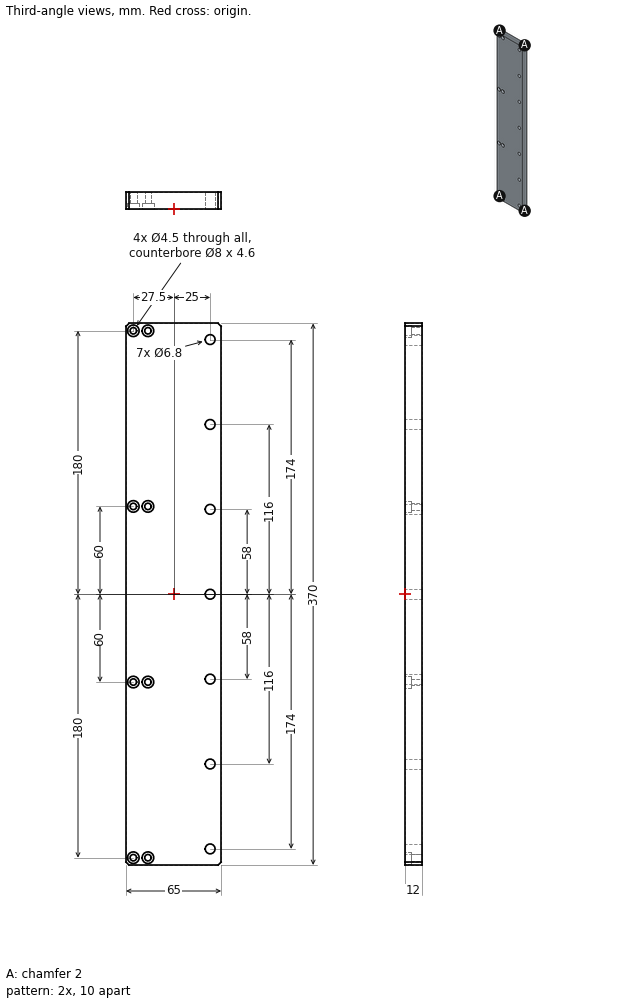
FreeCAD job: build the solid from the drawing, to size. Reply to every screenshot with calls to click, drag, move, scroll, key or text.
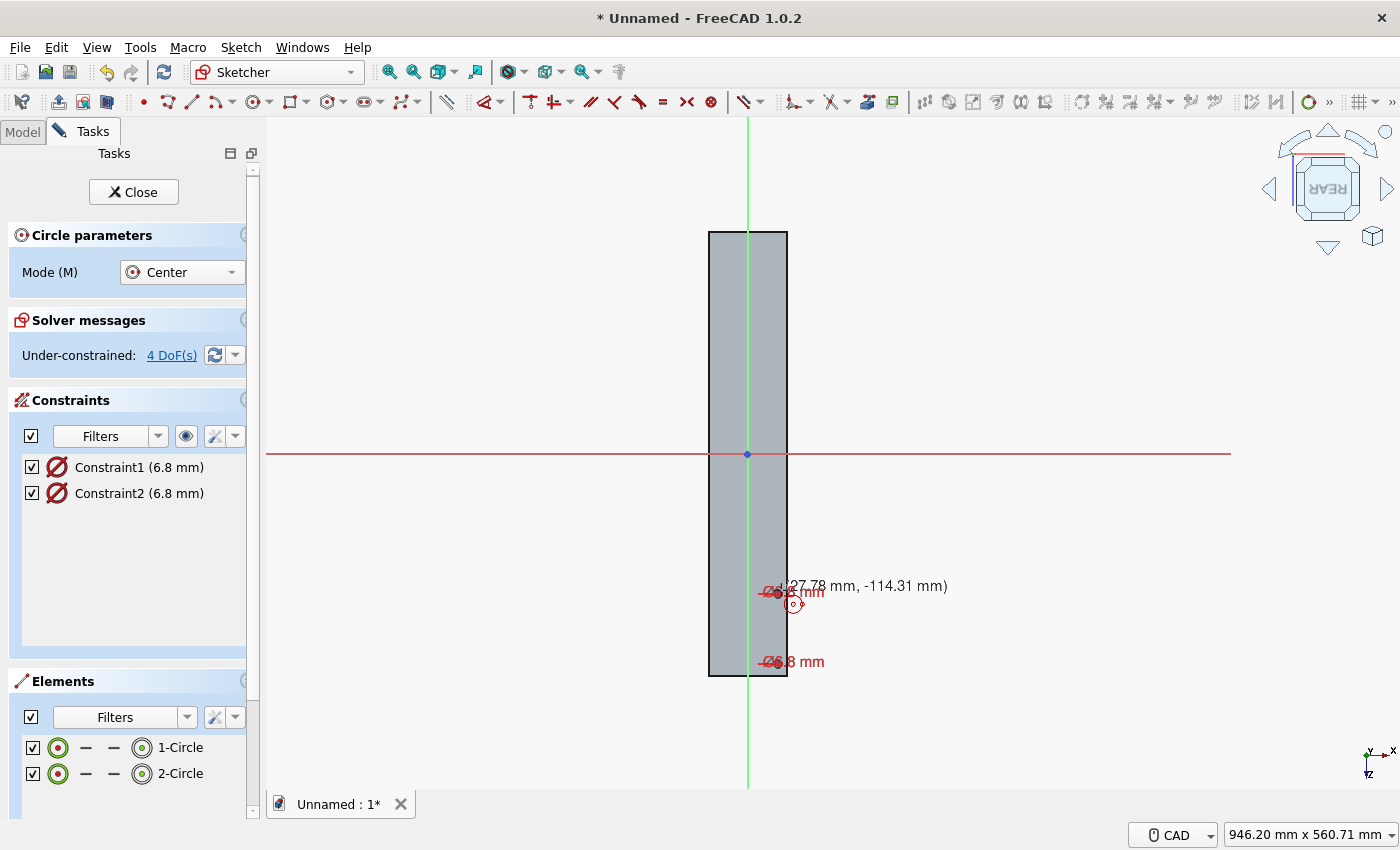
scroll(778, 524, up, 9)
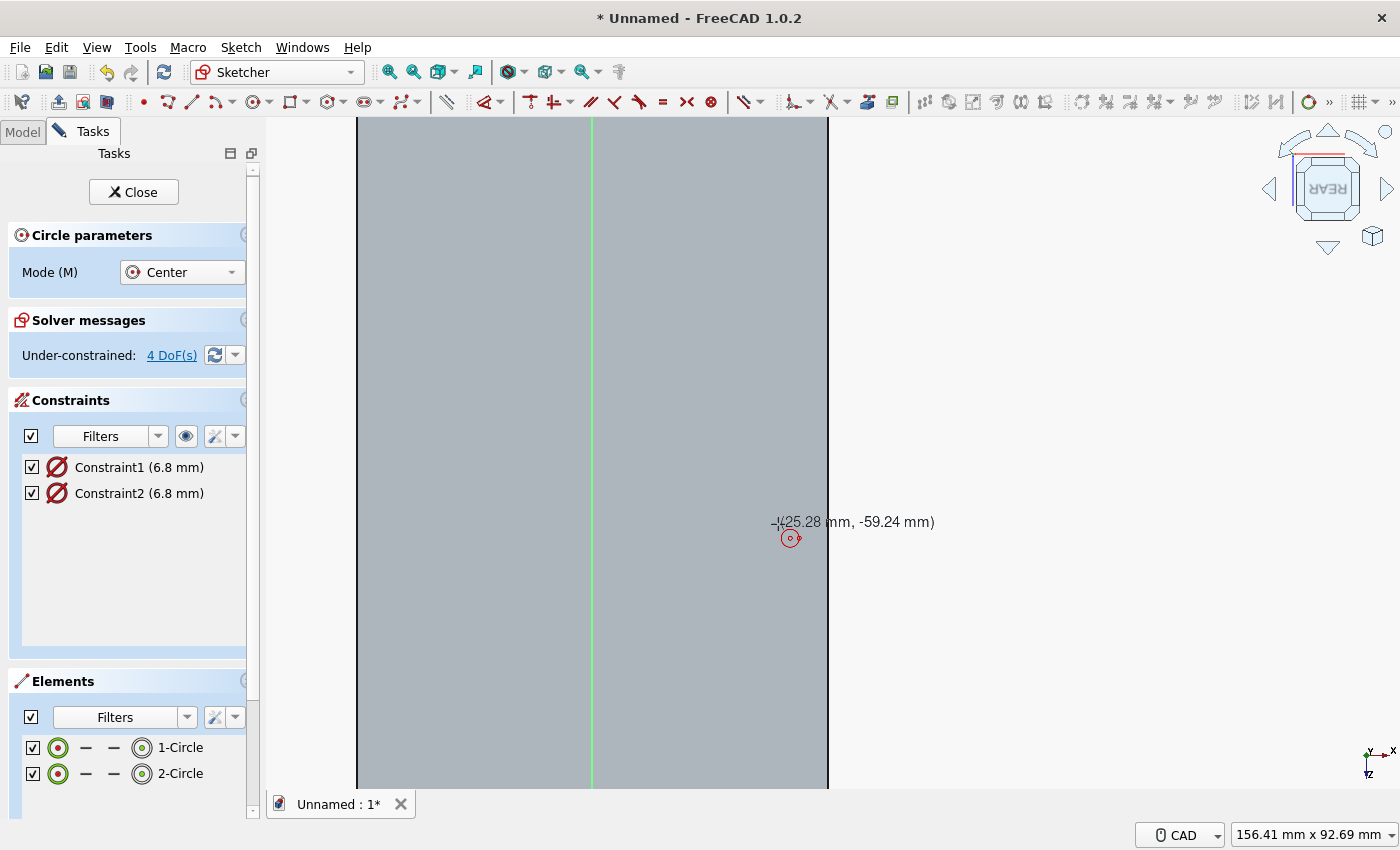
scroll(778, 523, down, 9)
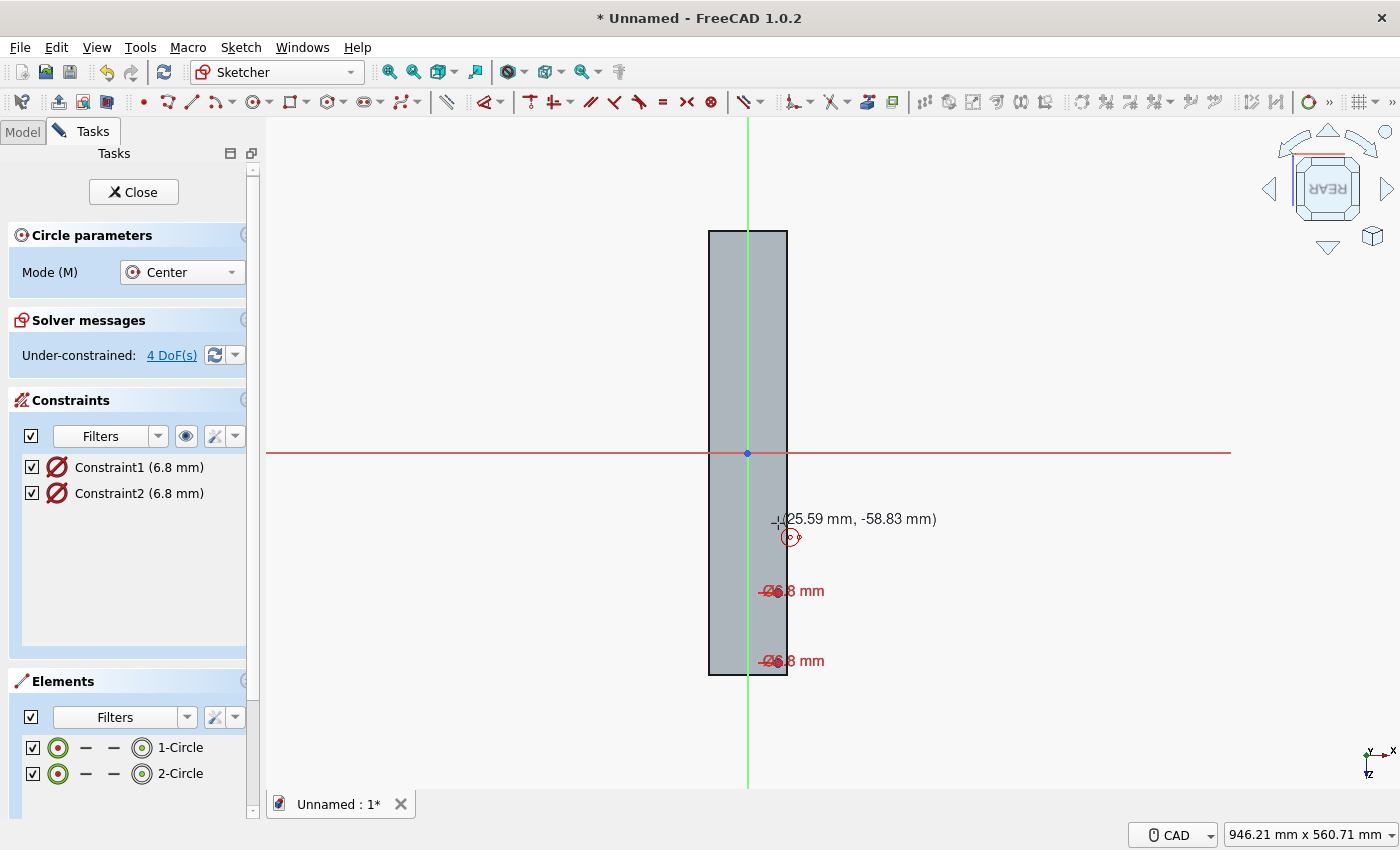
click(778, 523)
move(781, 520)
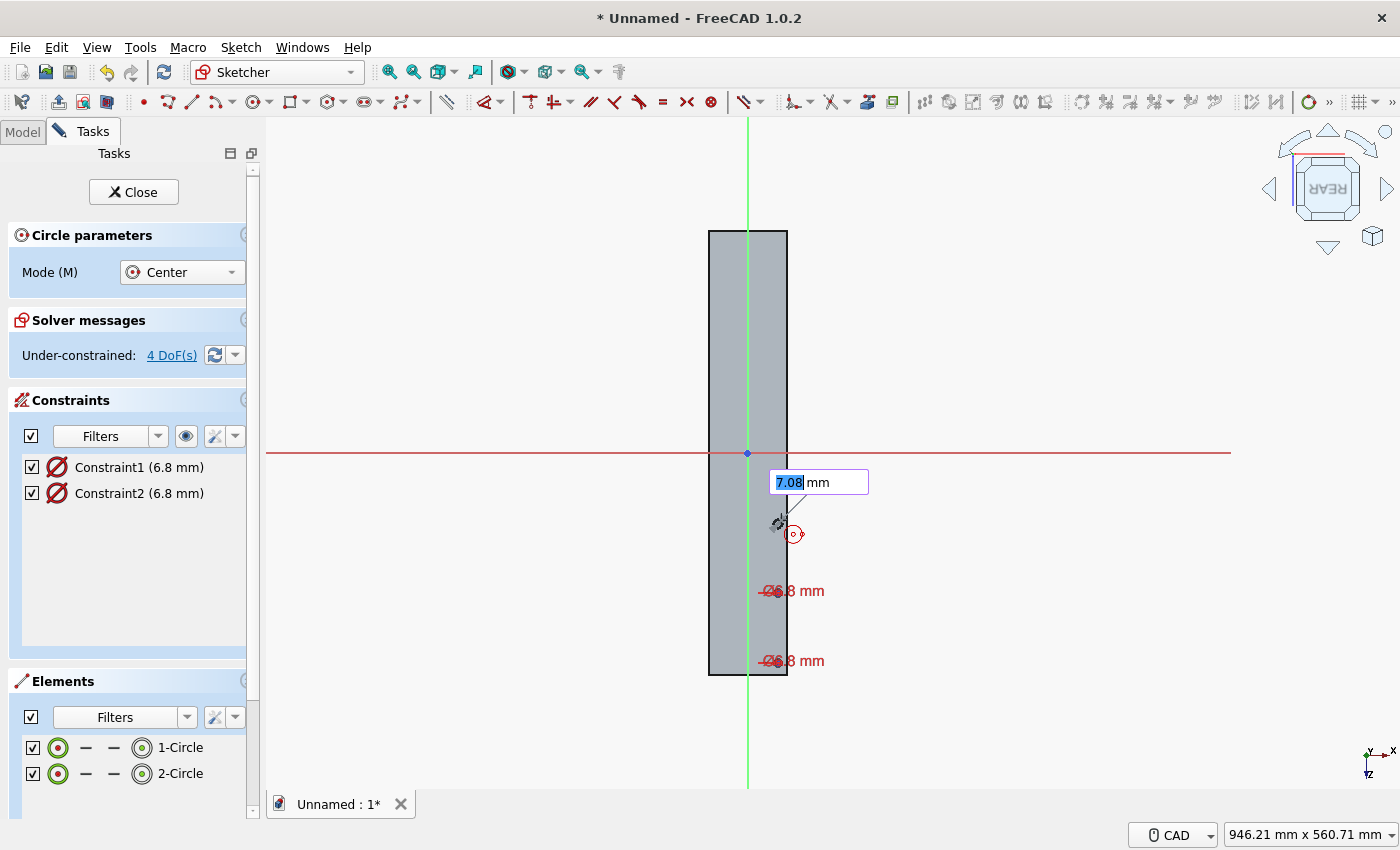
text(6.8)
key(Return)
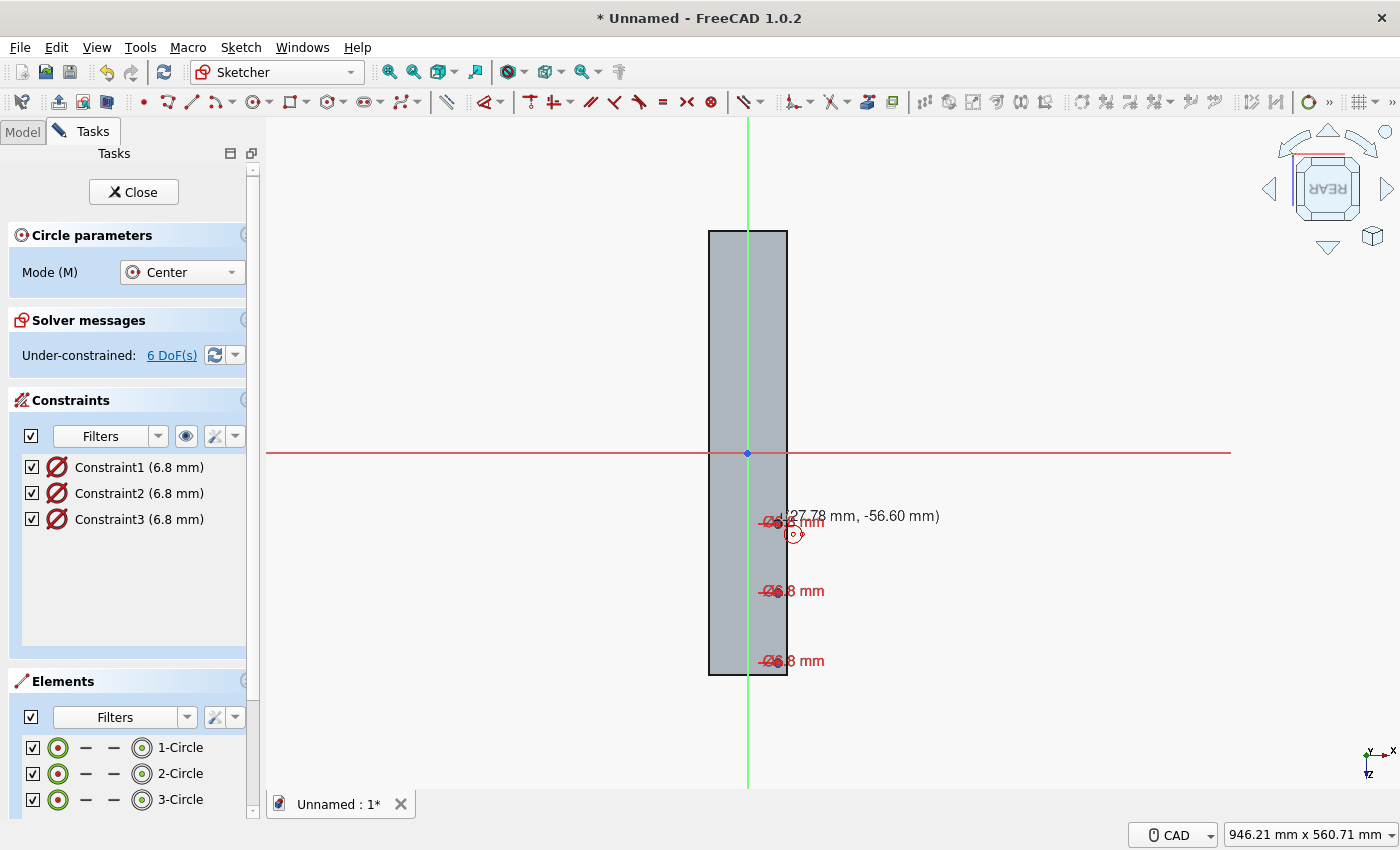
scroll(778, 453, up, 9)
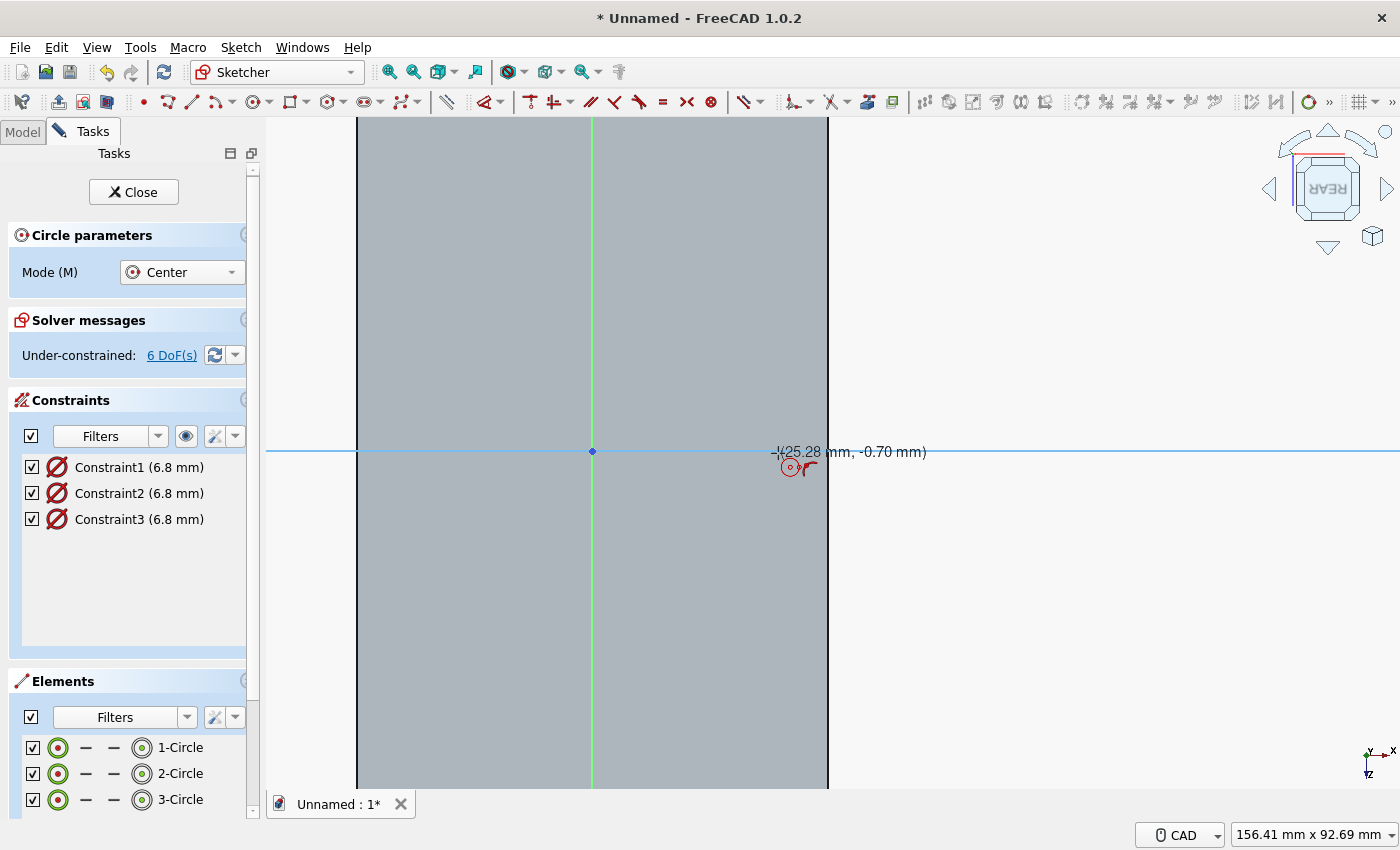
scroll(778, 453, down, 9)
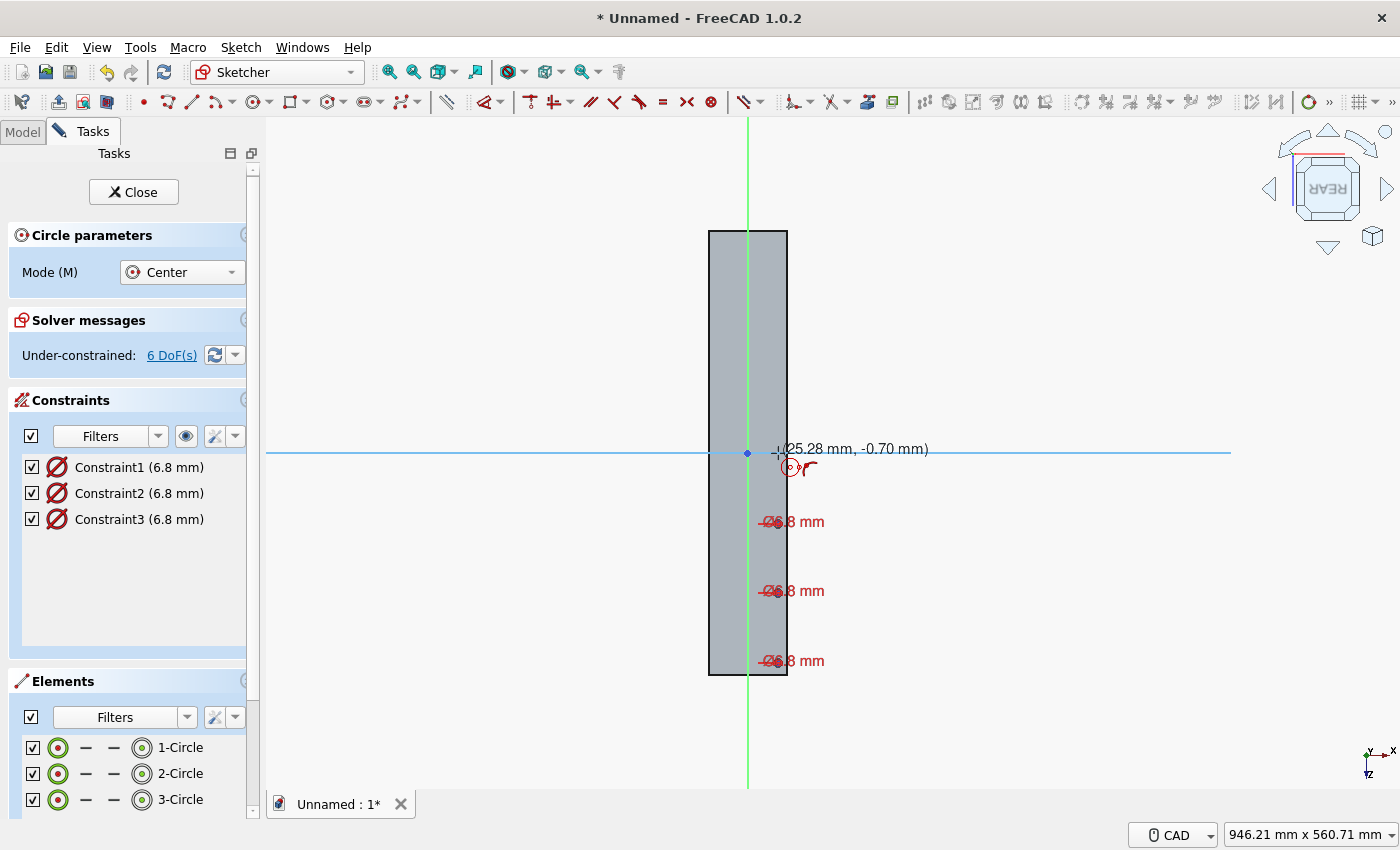
click(778, 453)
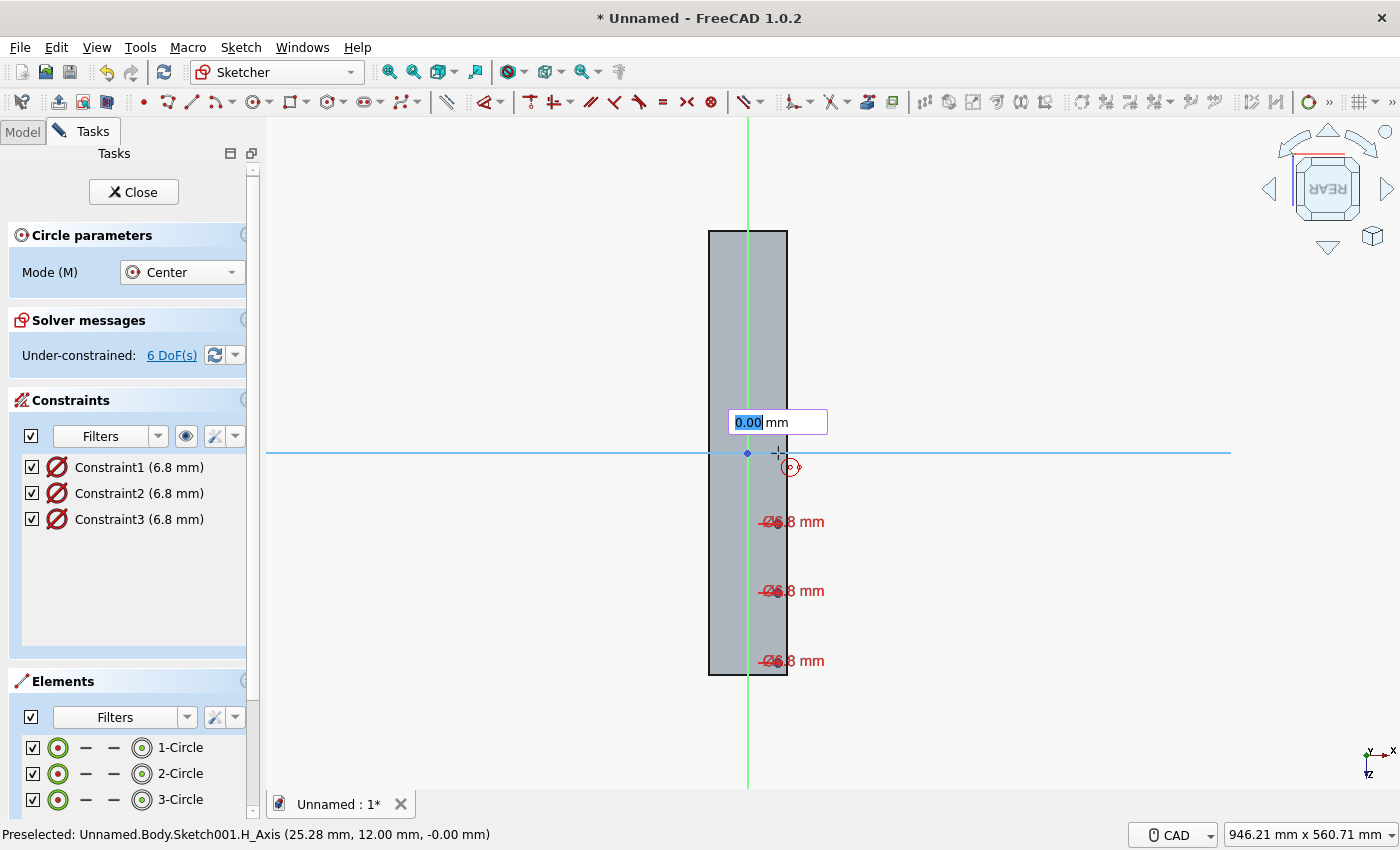
scroll(776, 457, up, 8)
move(776, 455)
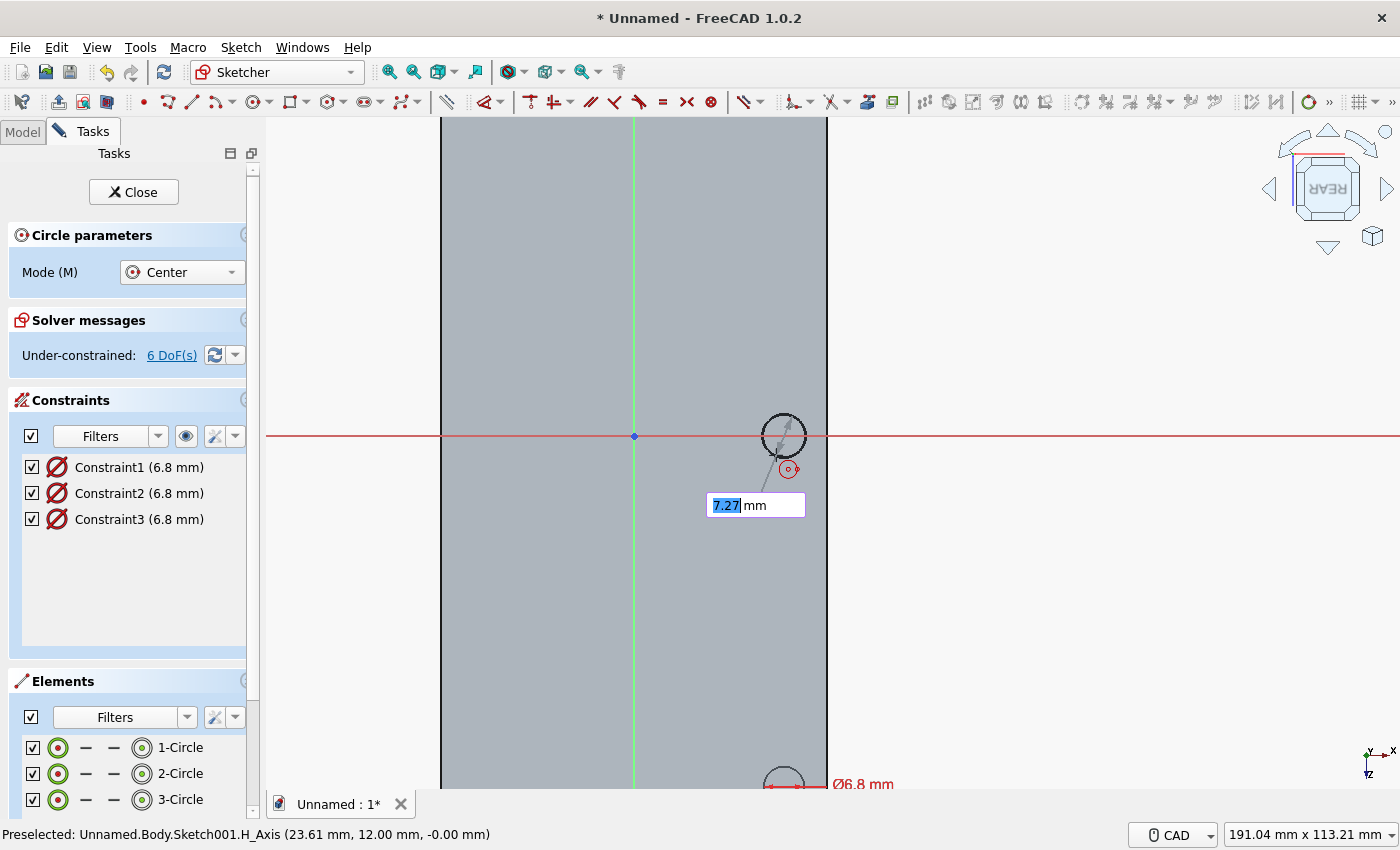
text(6.8)
key(Return)